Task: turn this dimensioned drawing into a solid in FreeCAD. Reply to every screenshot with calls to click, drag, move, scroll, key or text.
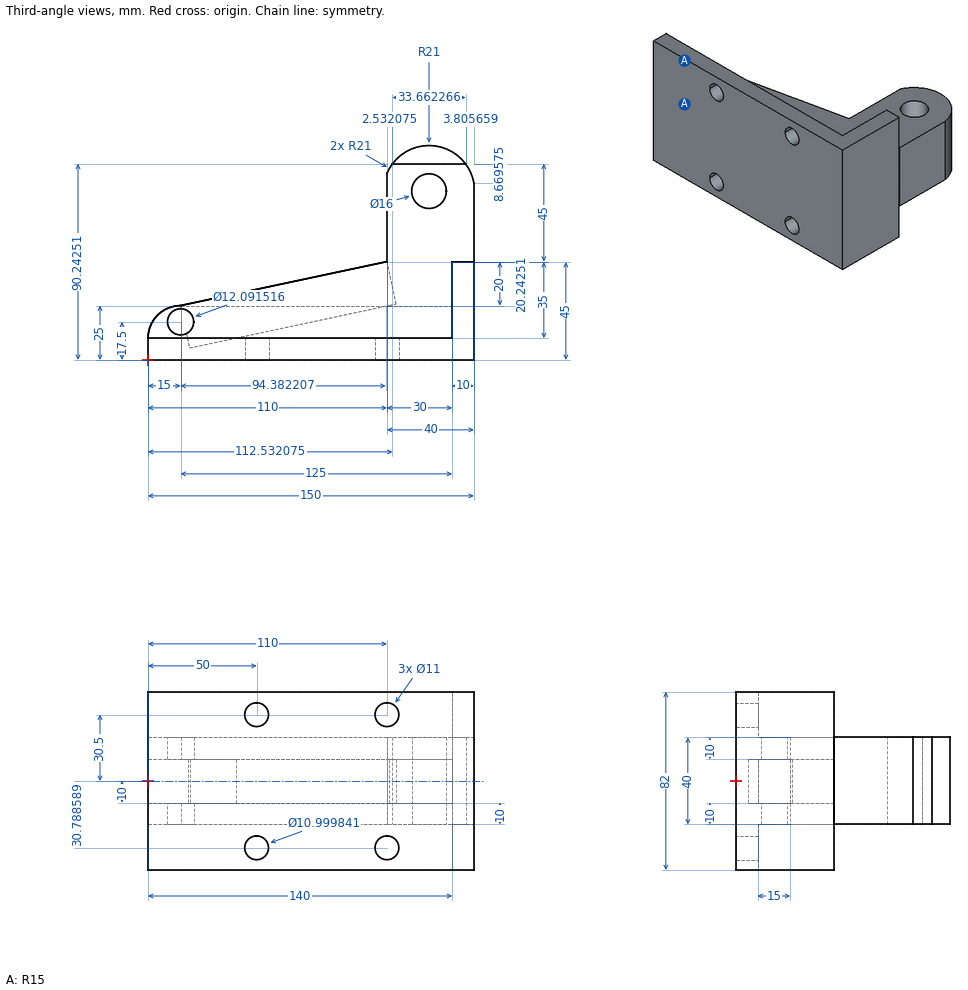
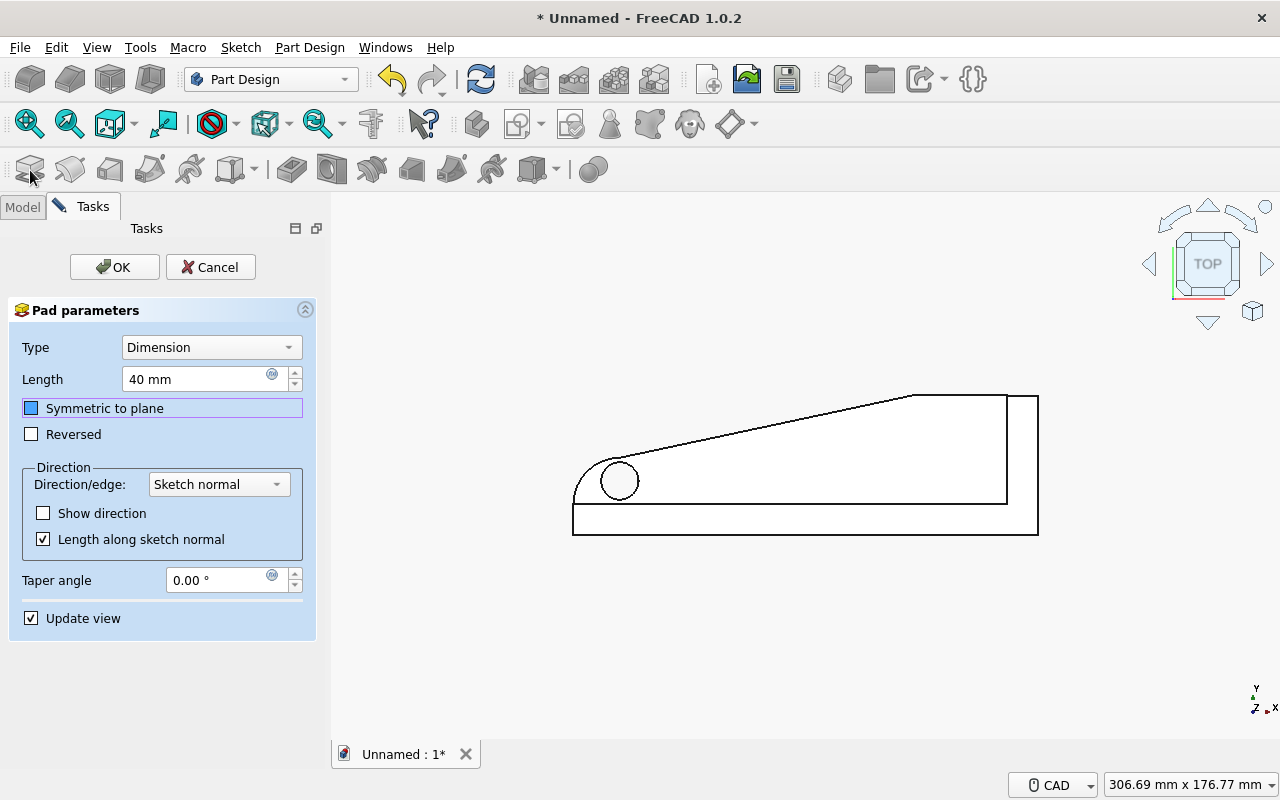
click(30, 434)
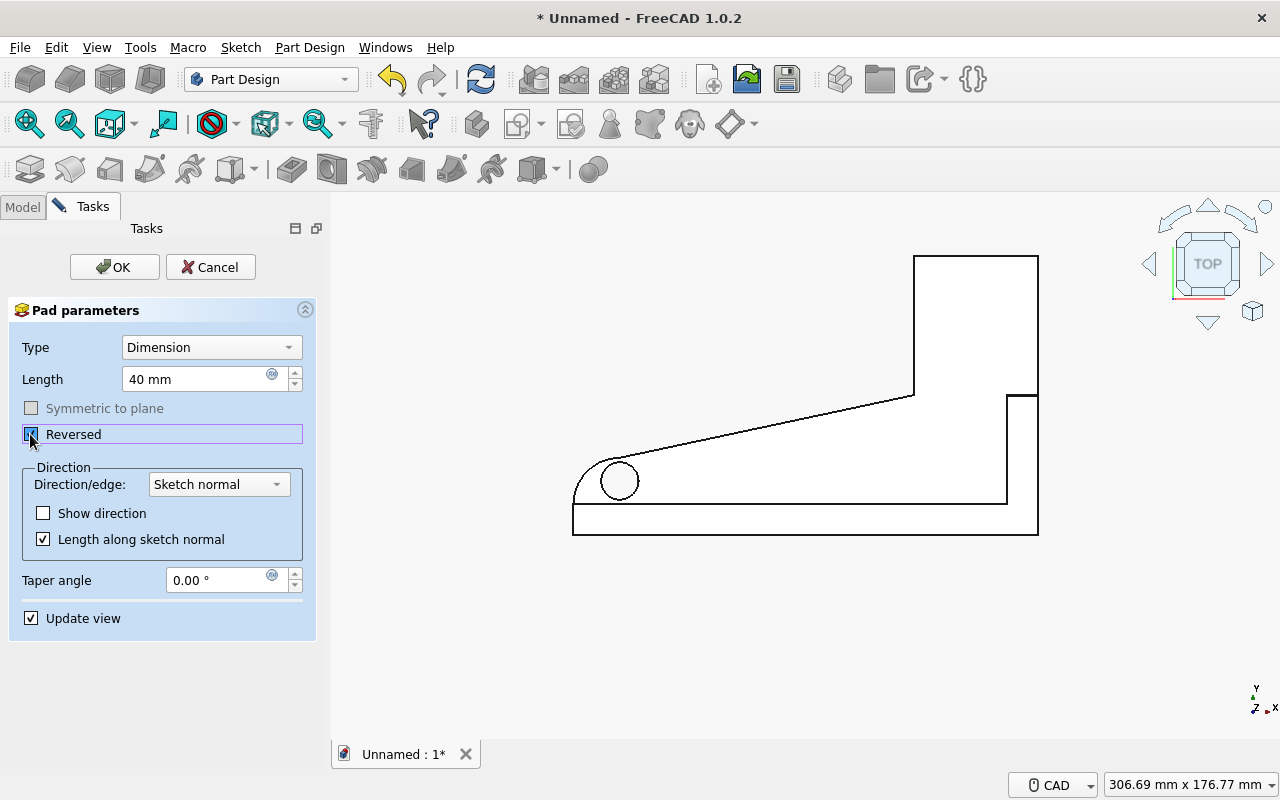
click(115, 267)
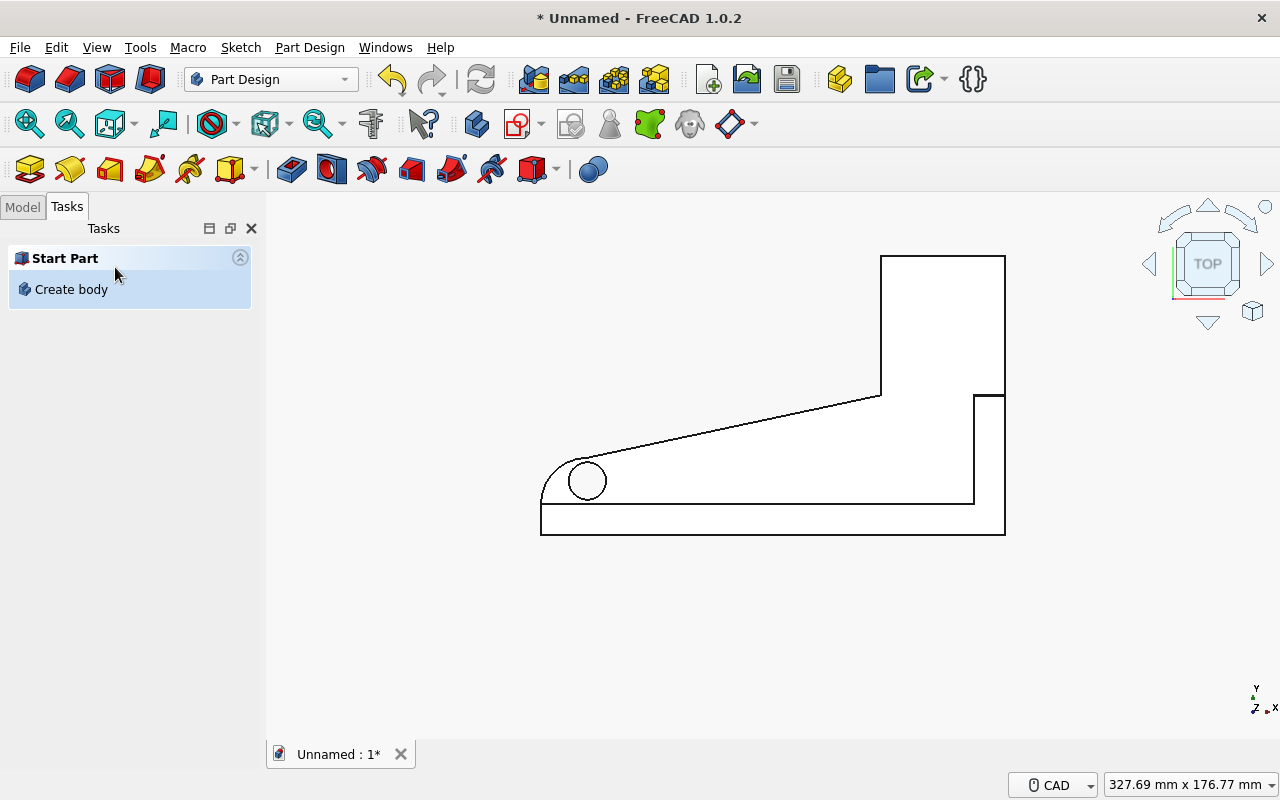
click(906, 450)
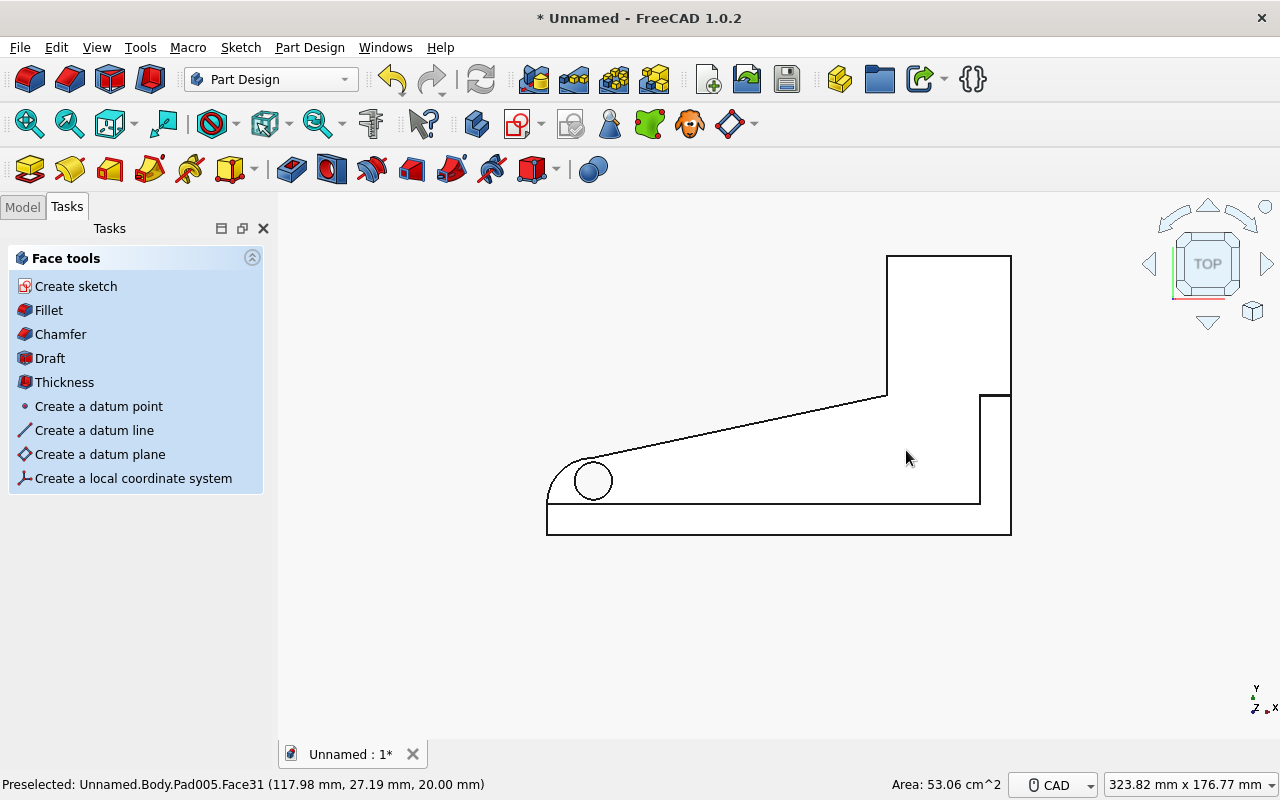
click(518, 124)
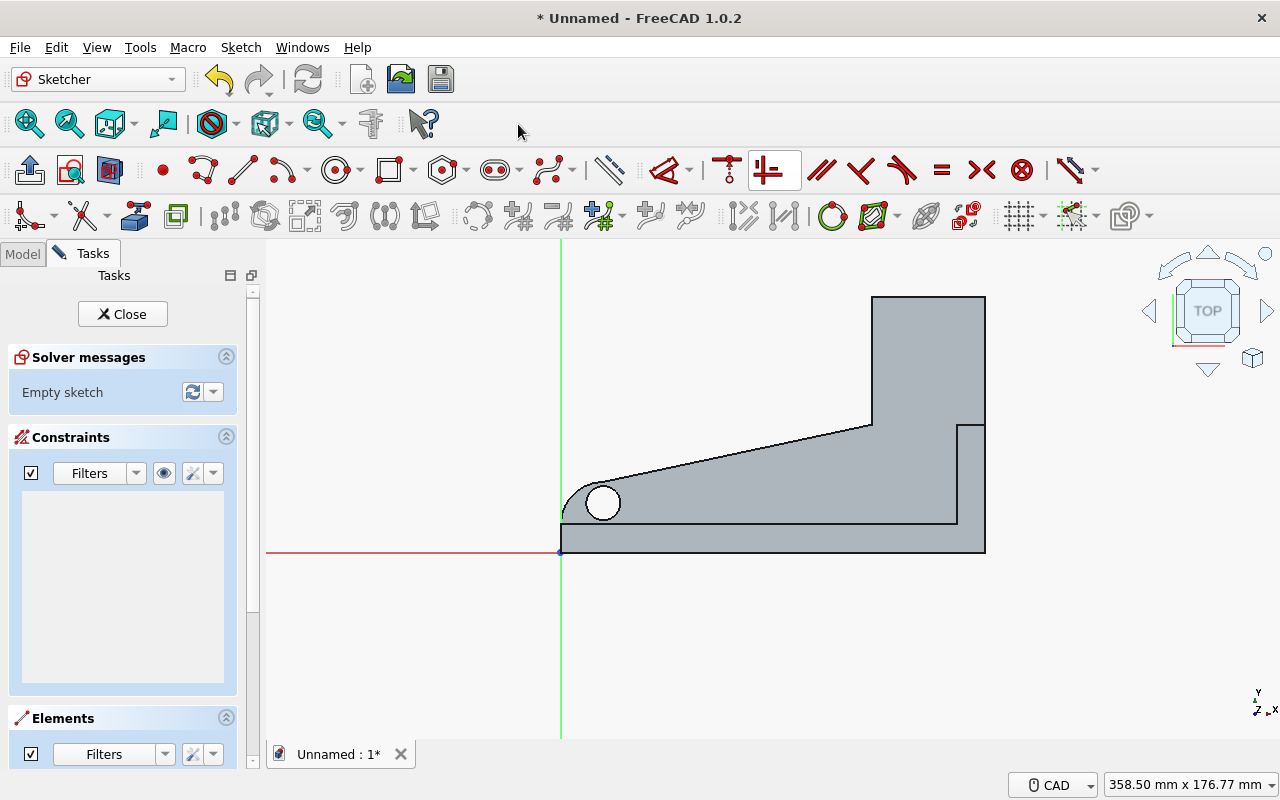
scroll(985, 285, up, 8)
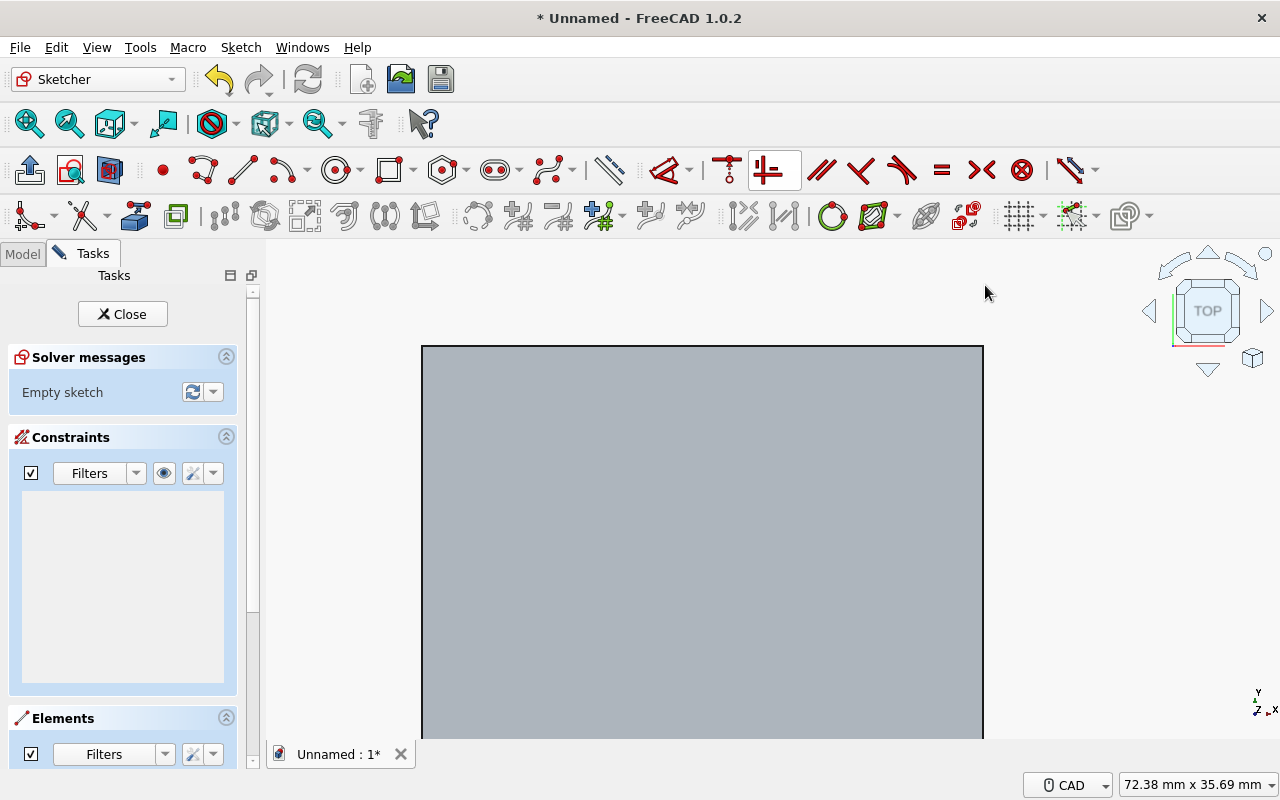
click(204, 170)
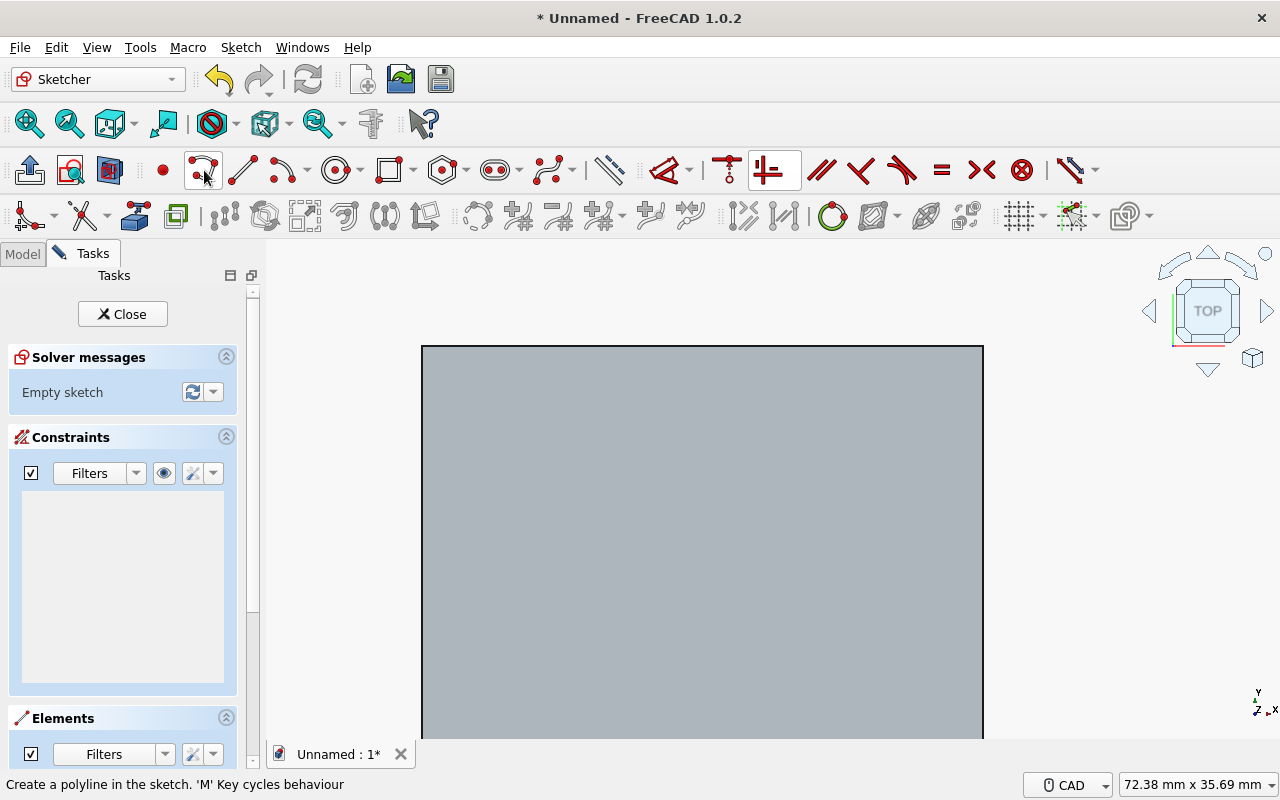
click(458, 346)
click(422, 346)
click(422, 408)
right_click(422, 408)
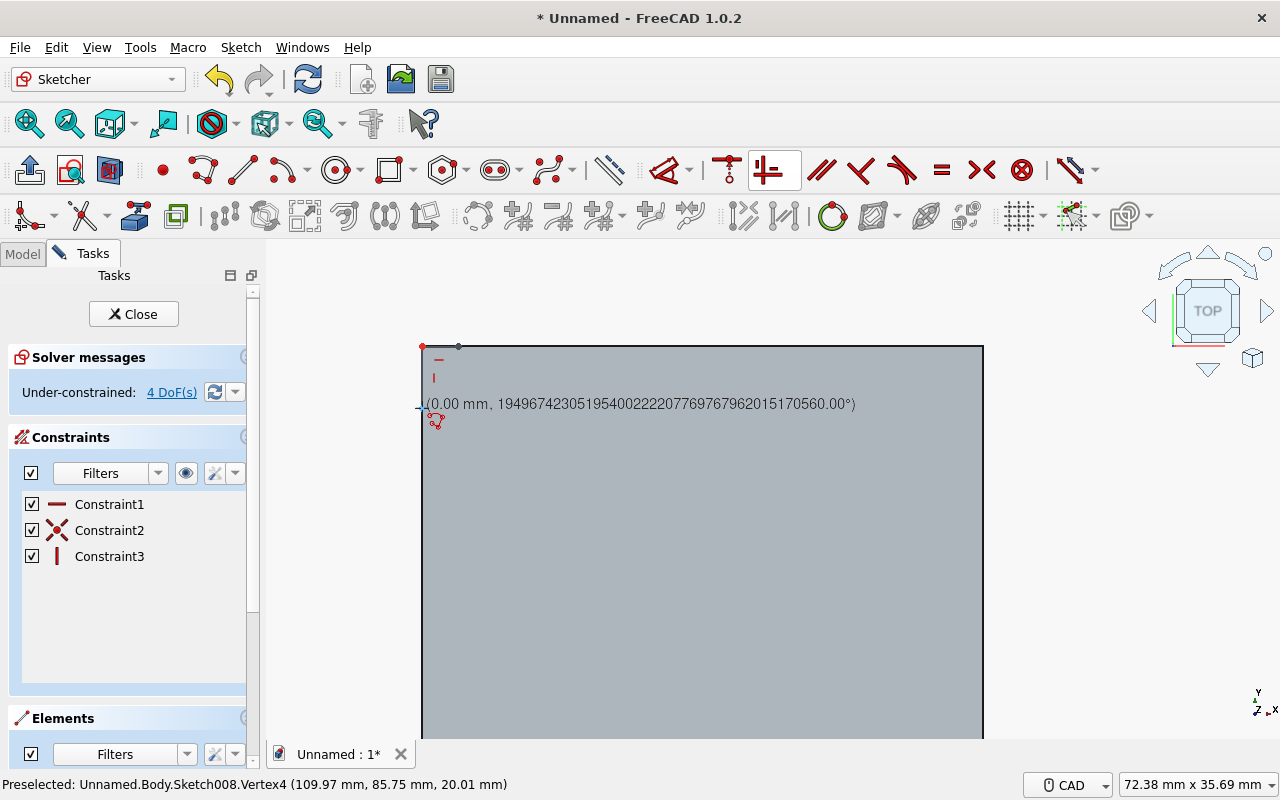
key(g)
key(3)
key(a)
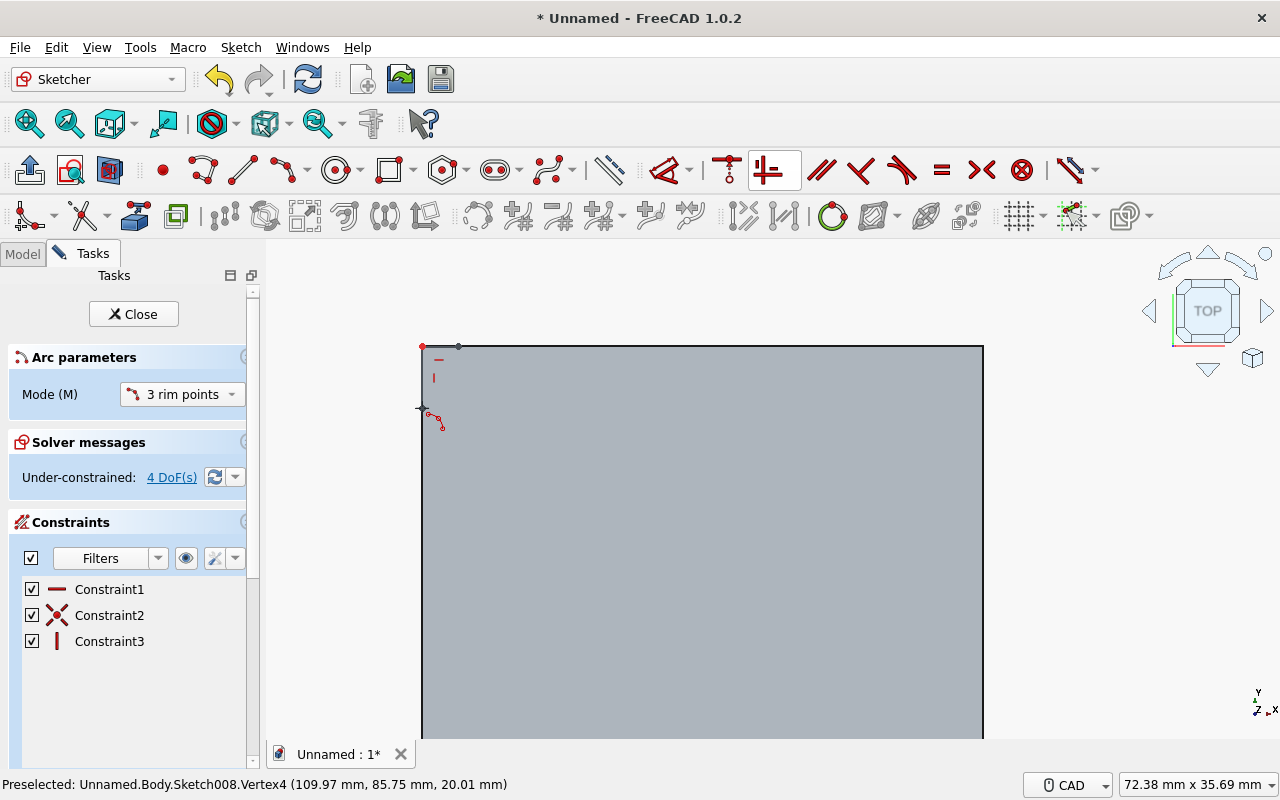
click(422, 409)
click(458, 347)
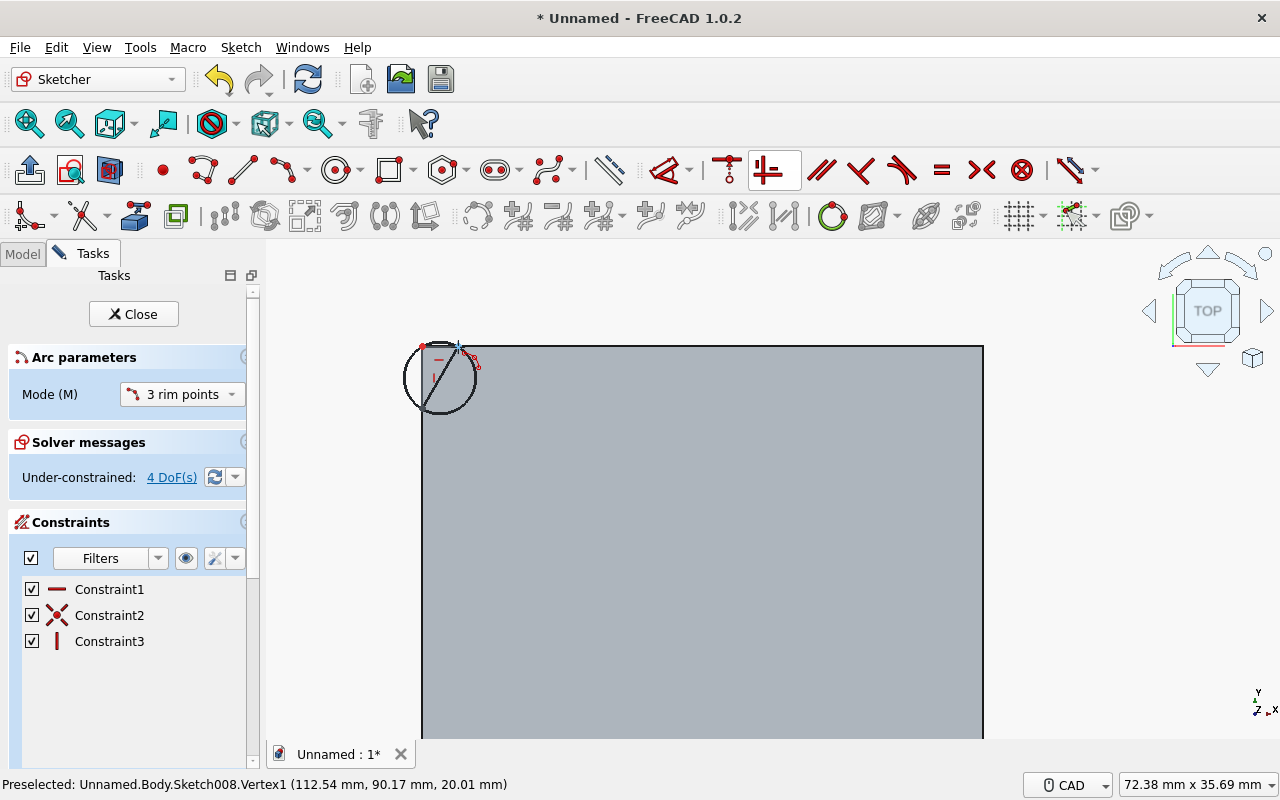
scroll(438, 376, up, 10)